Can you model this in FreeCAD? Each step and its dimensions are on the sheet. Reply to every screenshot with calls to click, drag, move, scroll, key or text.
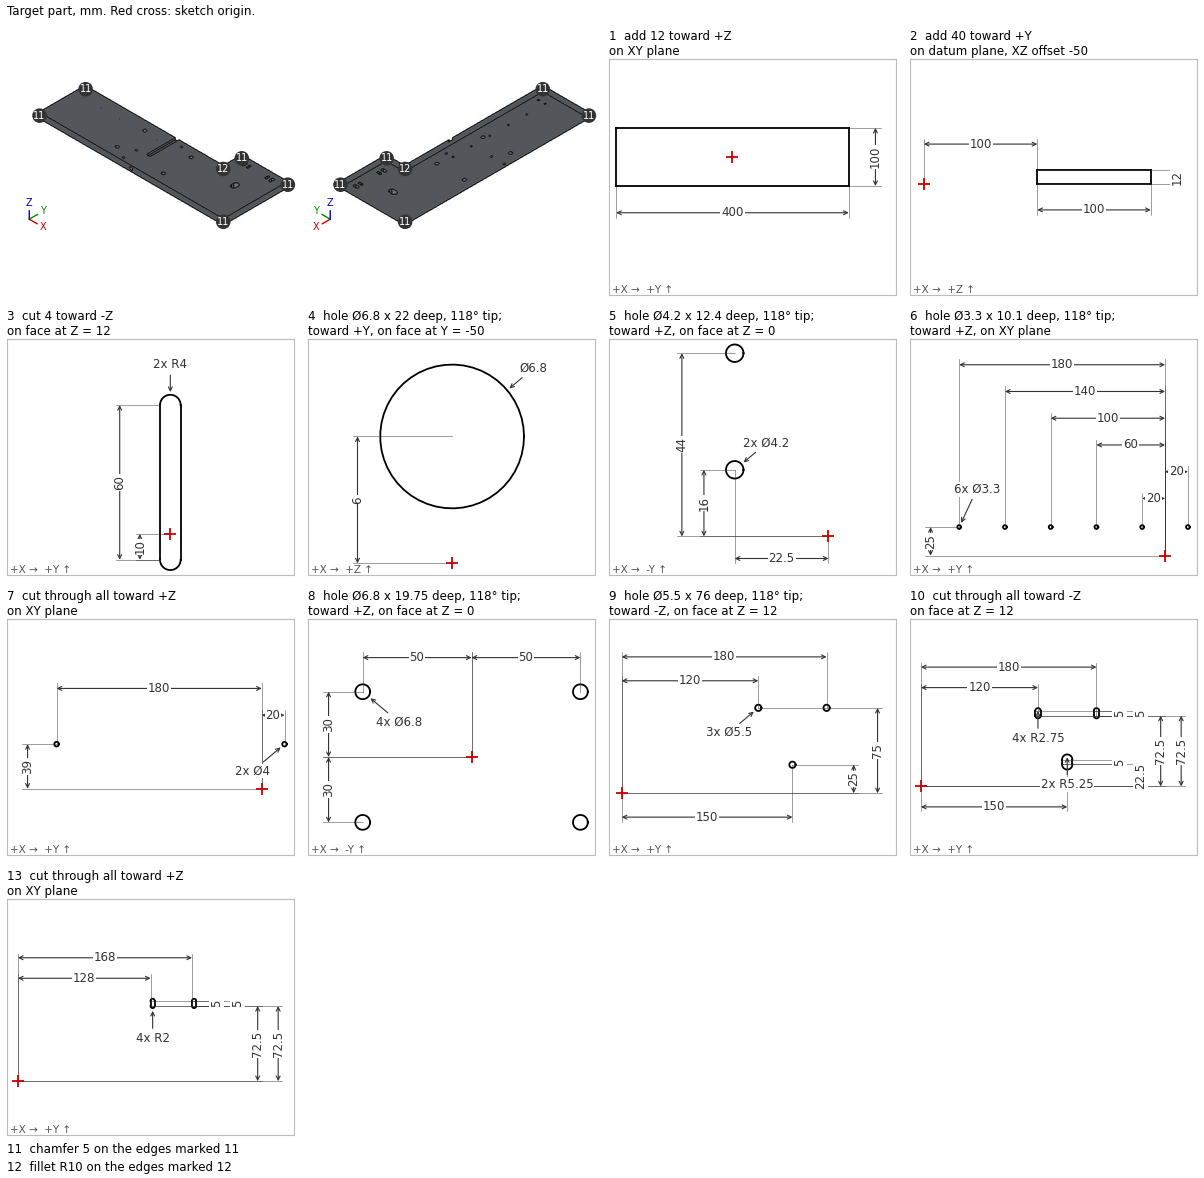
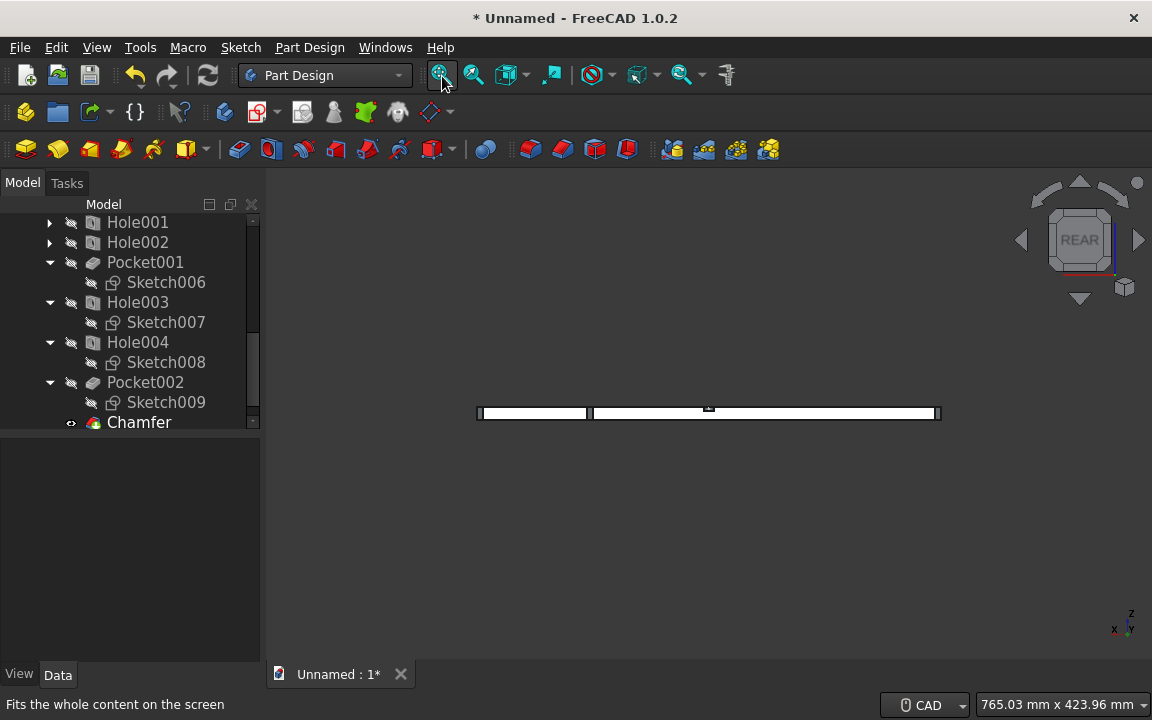
scroll(593, 412, up, 6)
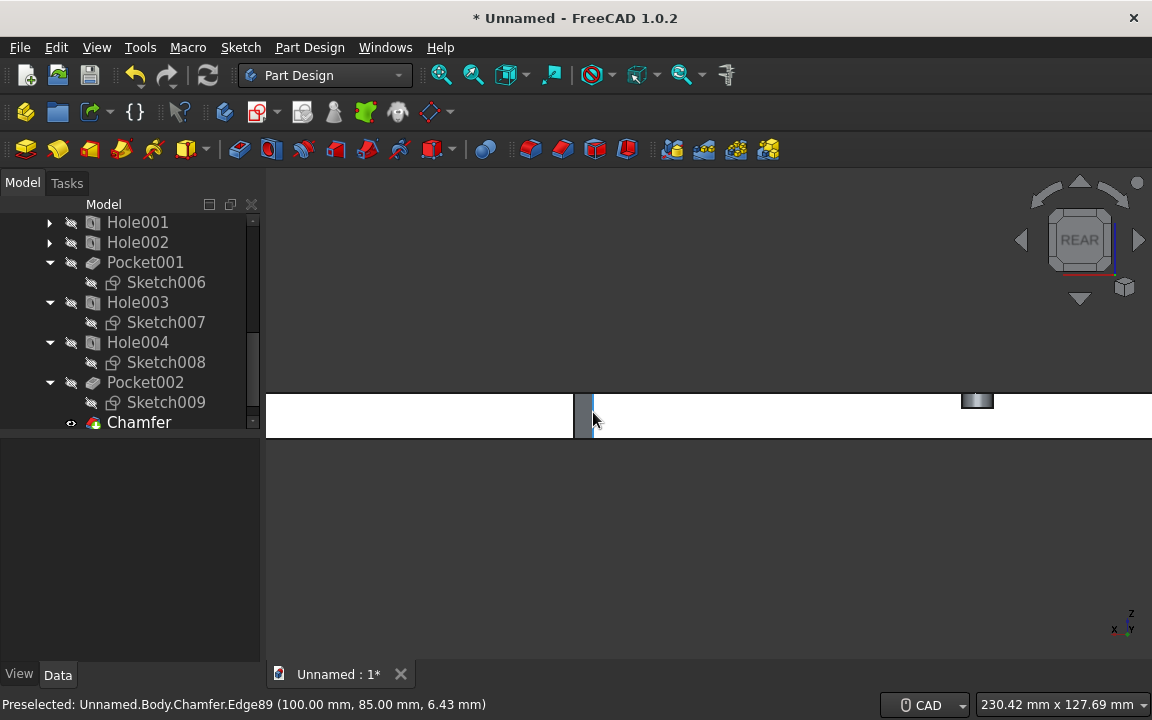
click(442, 76)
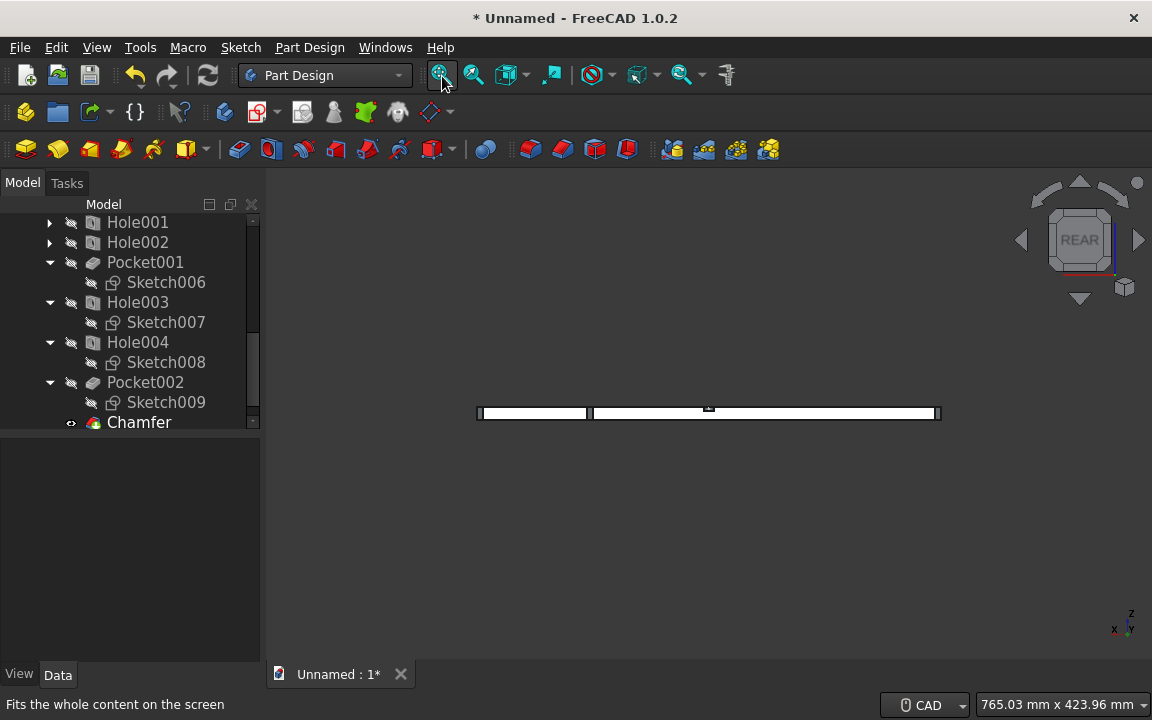
key(6)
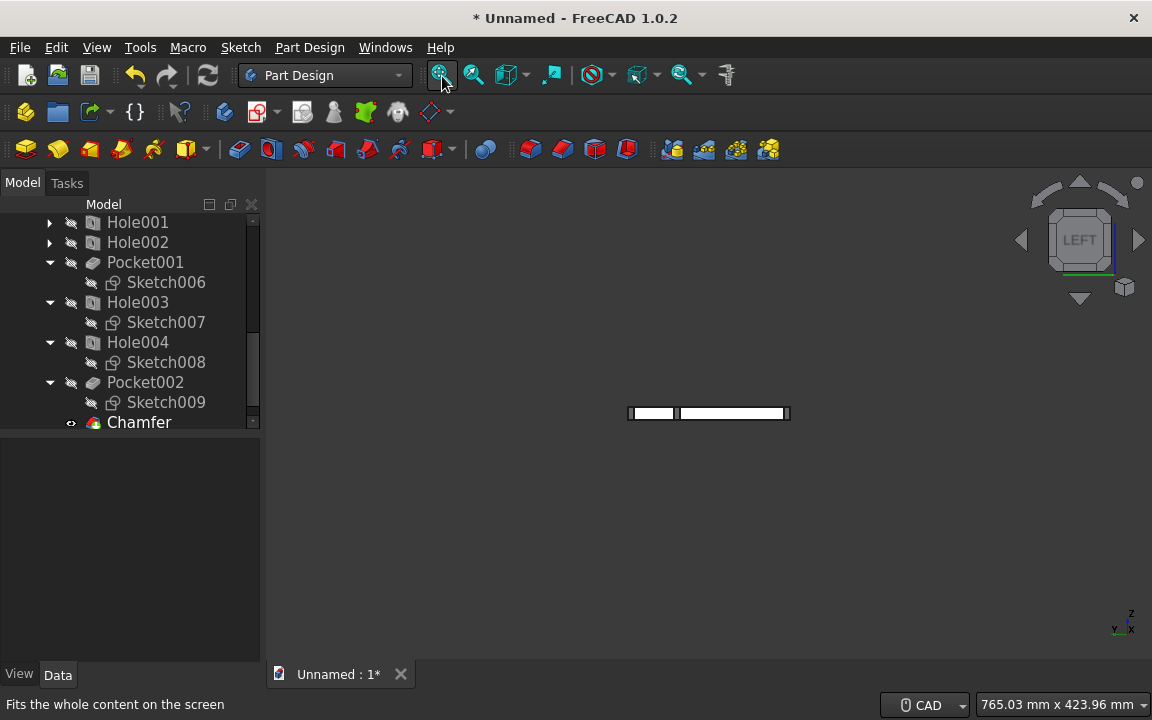
click(442, 76)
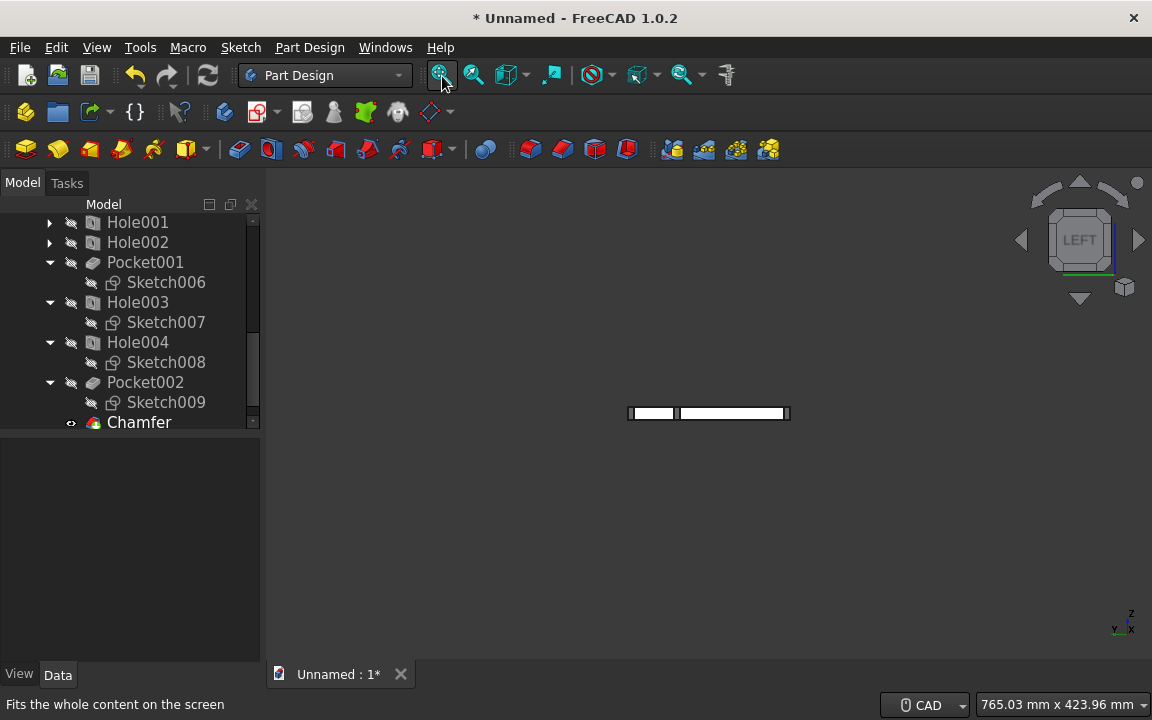
scroll(674, 412, up, 6)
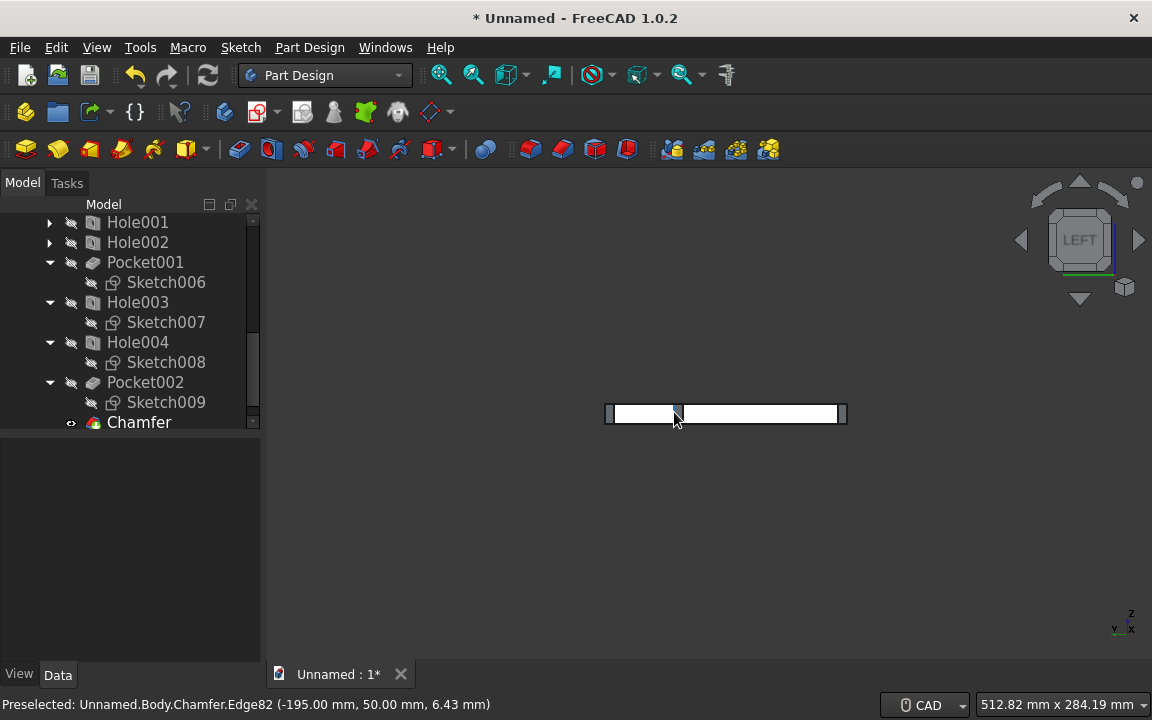
click(442, 76)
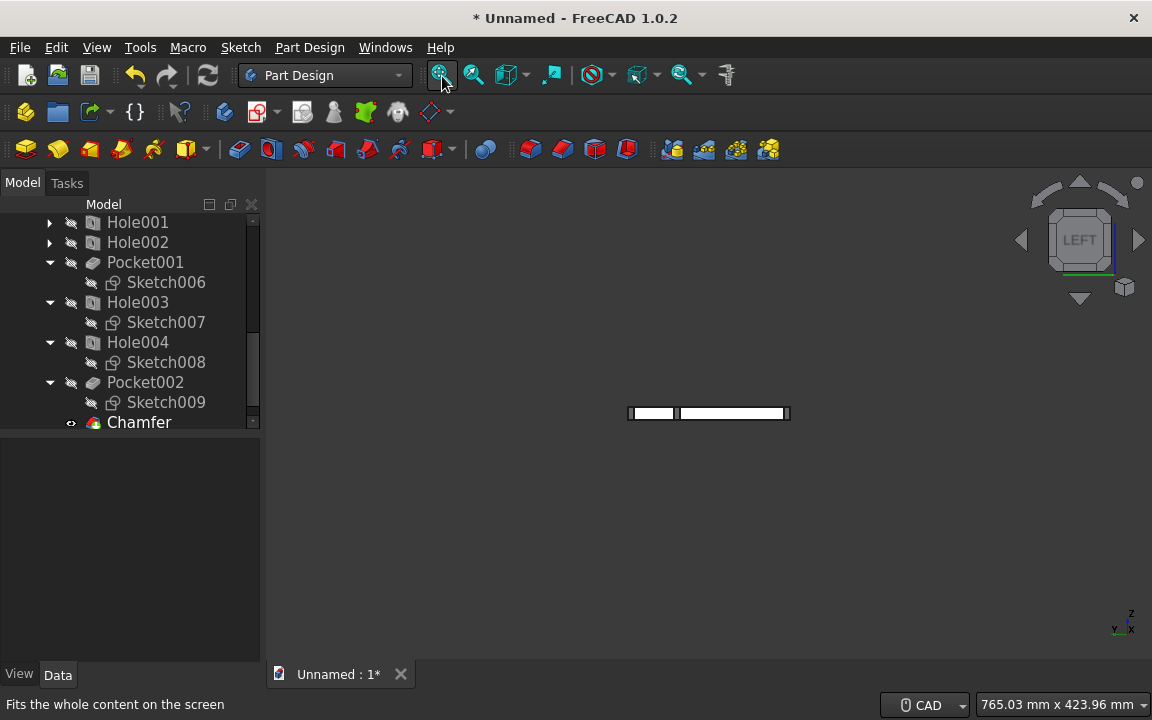
key(v)
key(3)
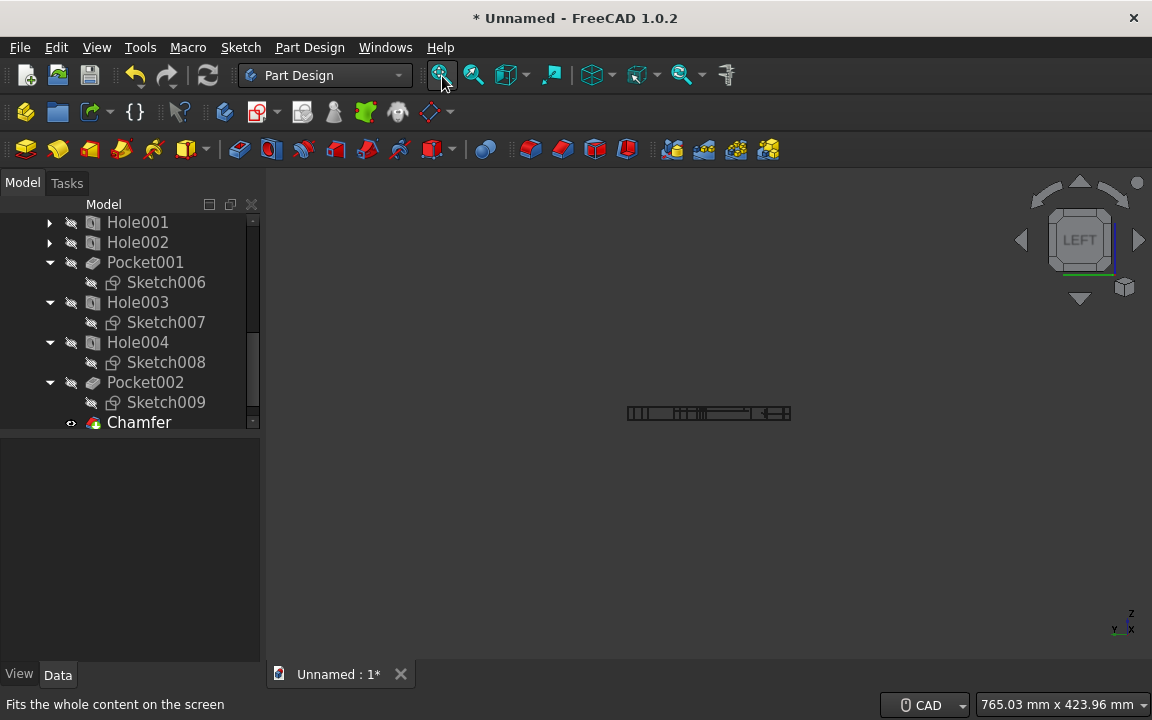
key(0)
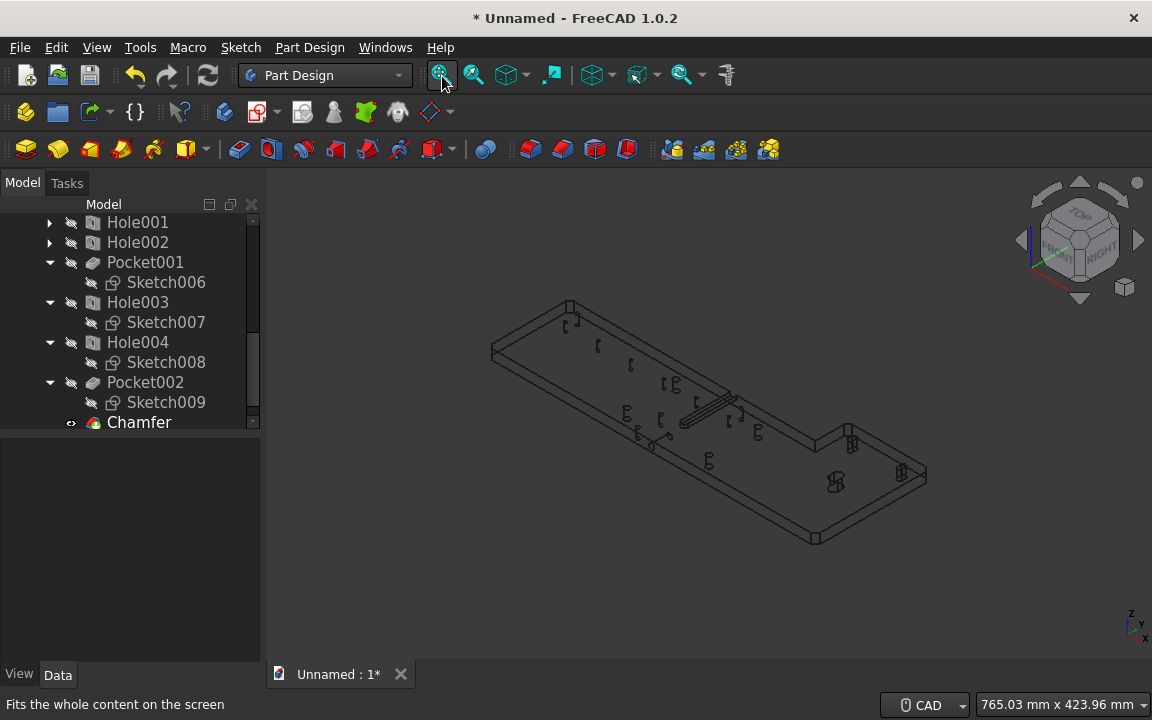
click(815, 446)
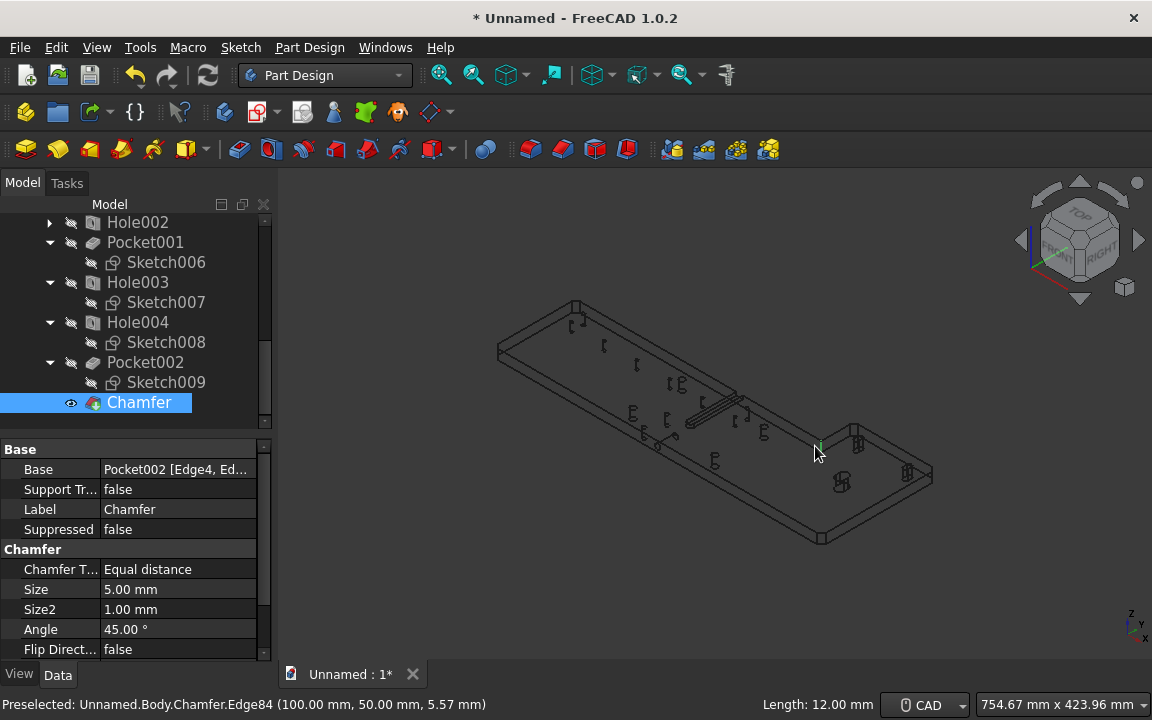
key(v)
key(1)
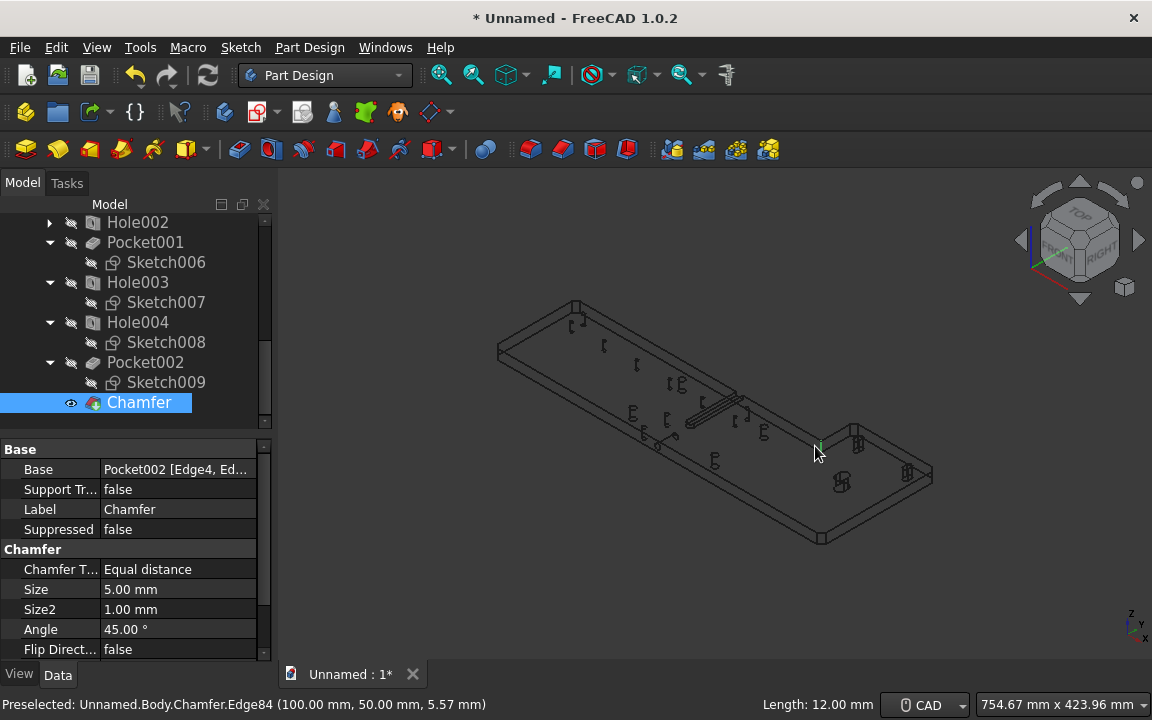
click(532, 150)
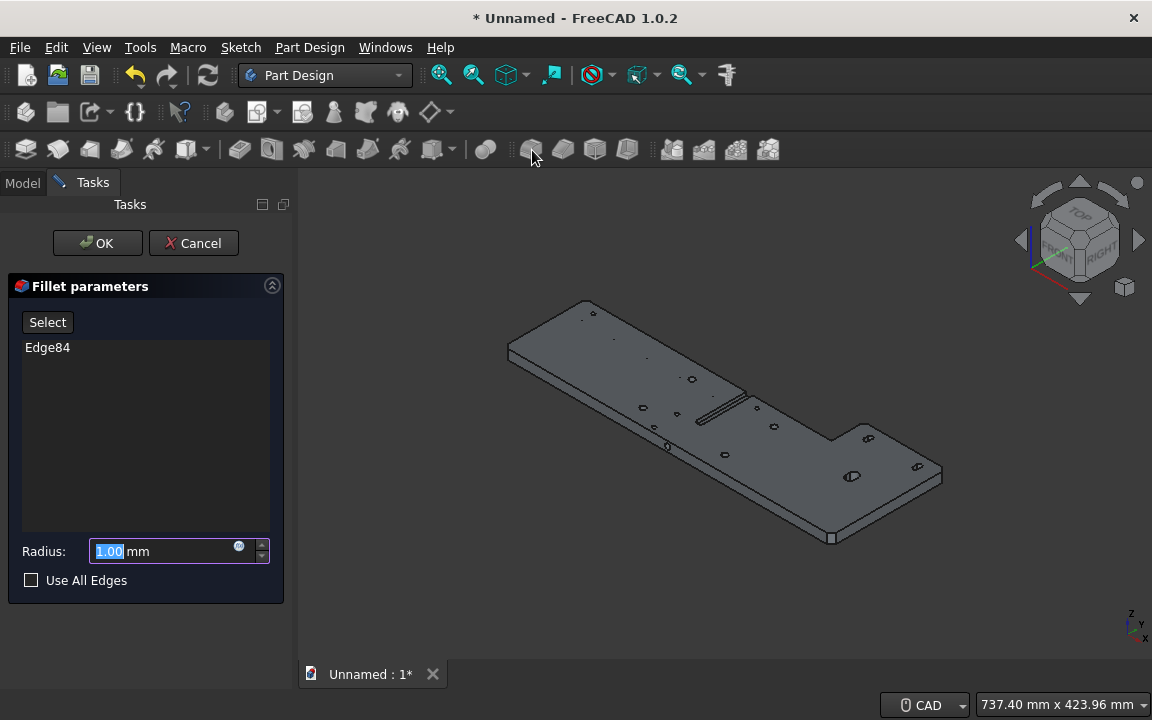
text(10)
key(Tab)